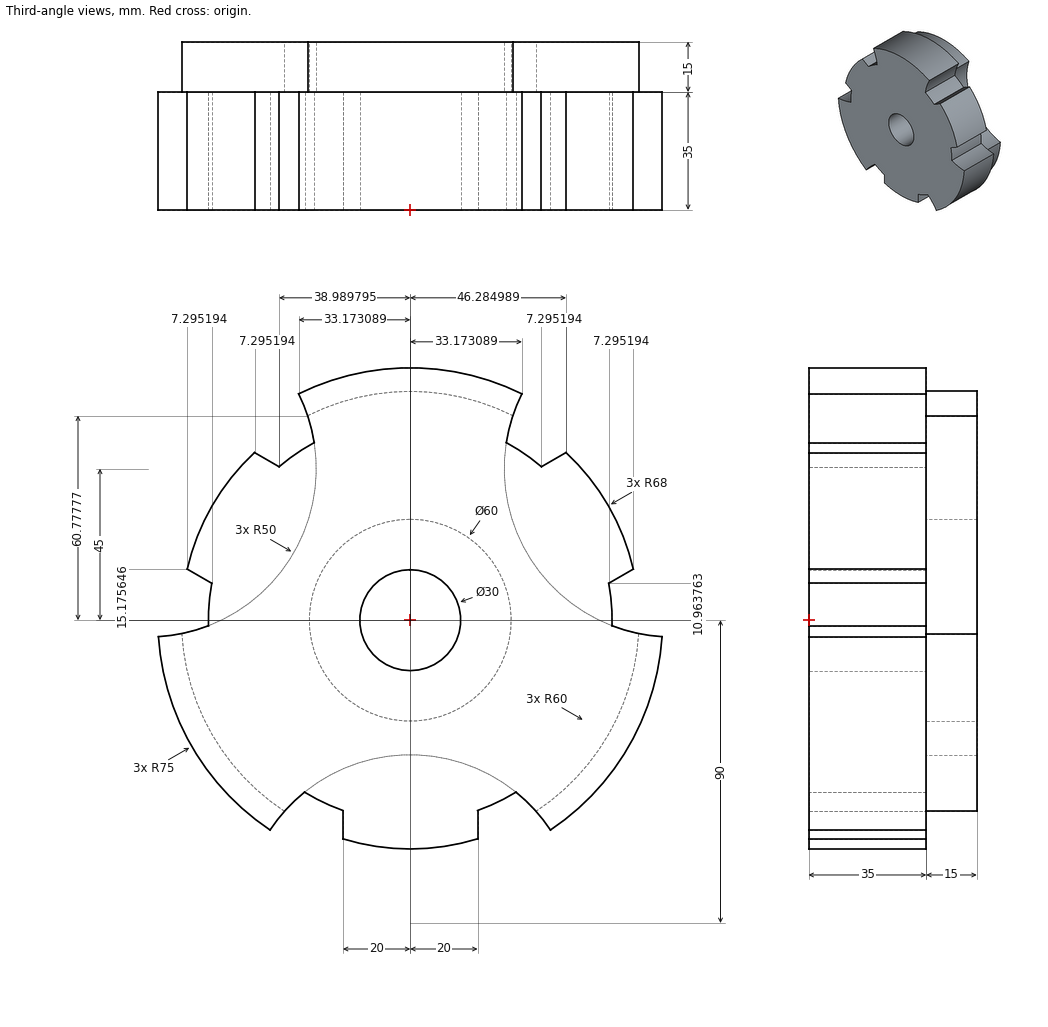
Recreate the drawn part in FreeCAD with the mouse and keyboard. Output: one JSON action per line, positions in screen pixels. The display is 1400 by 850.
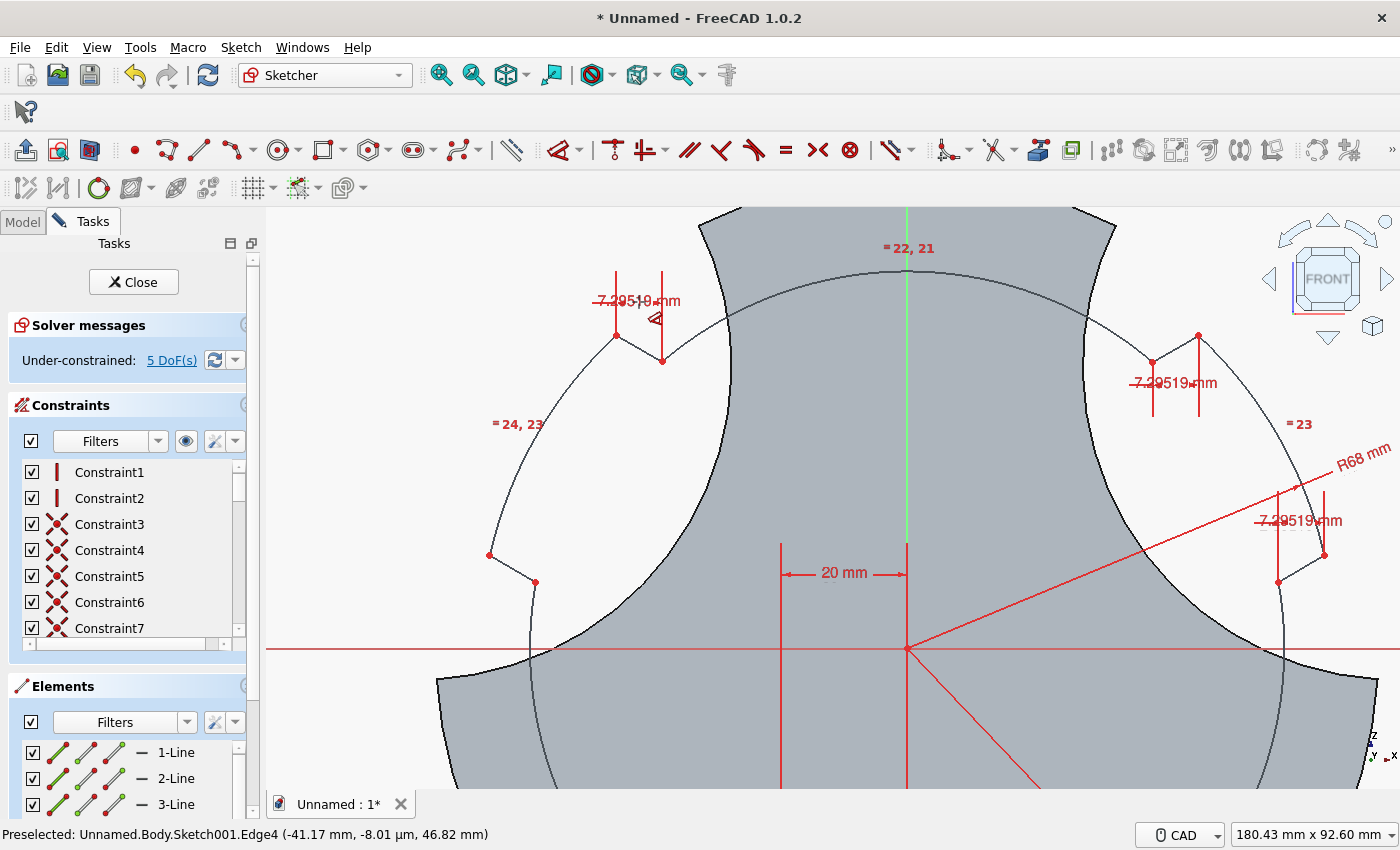
{"action": "left_click", "coordinate": [504, 564]}
{"action": "left_click", "coordinate": [513, 522]}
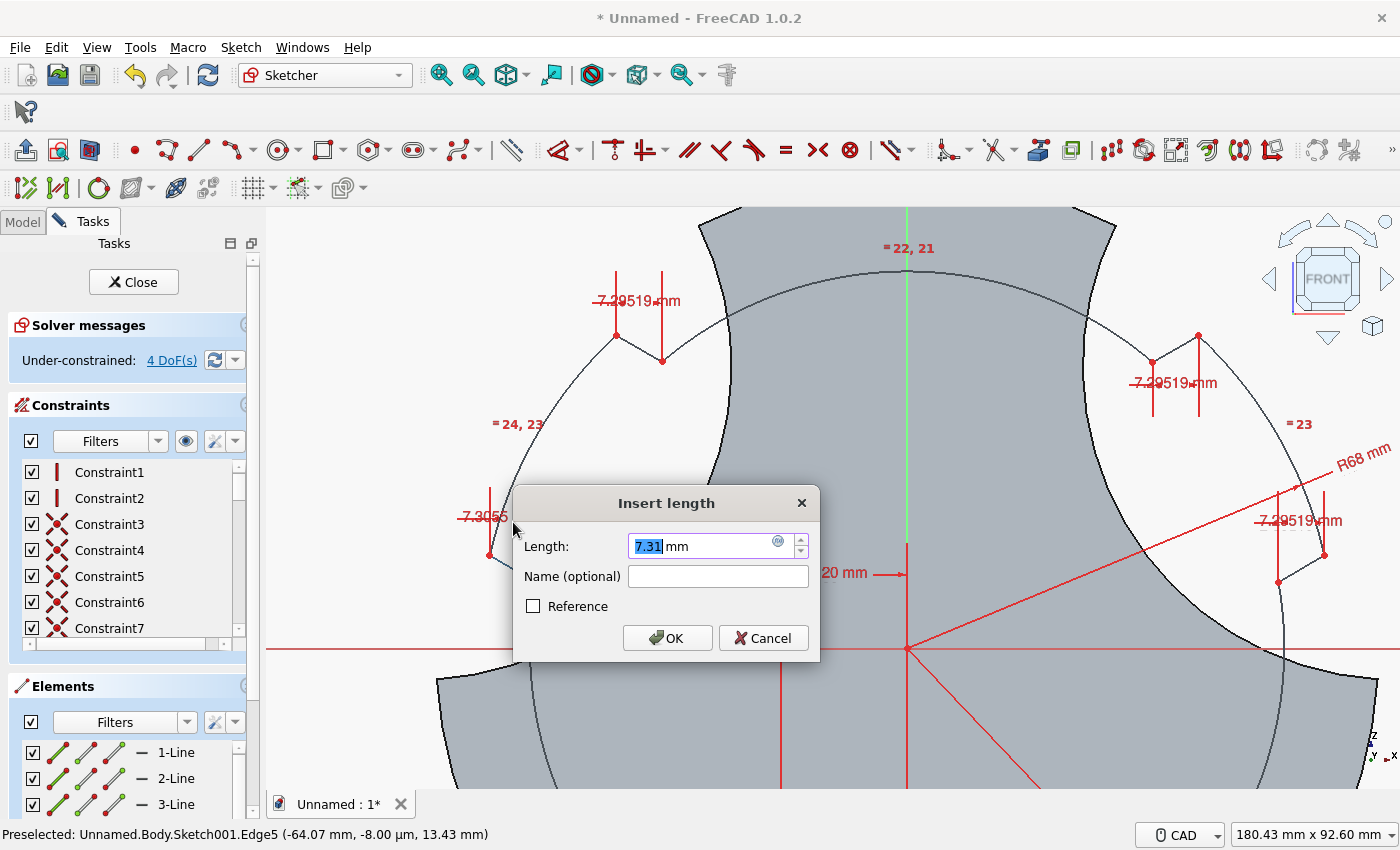
{"action": "type", "text": "7.295194"}
{"action": "key", "text": "Return"}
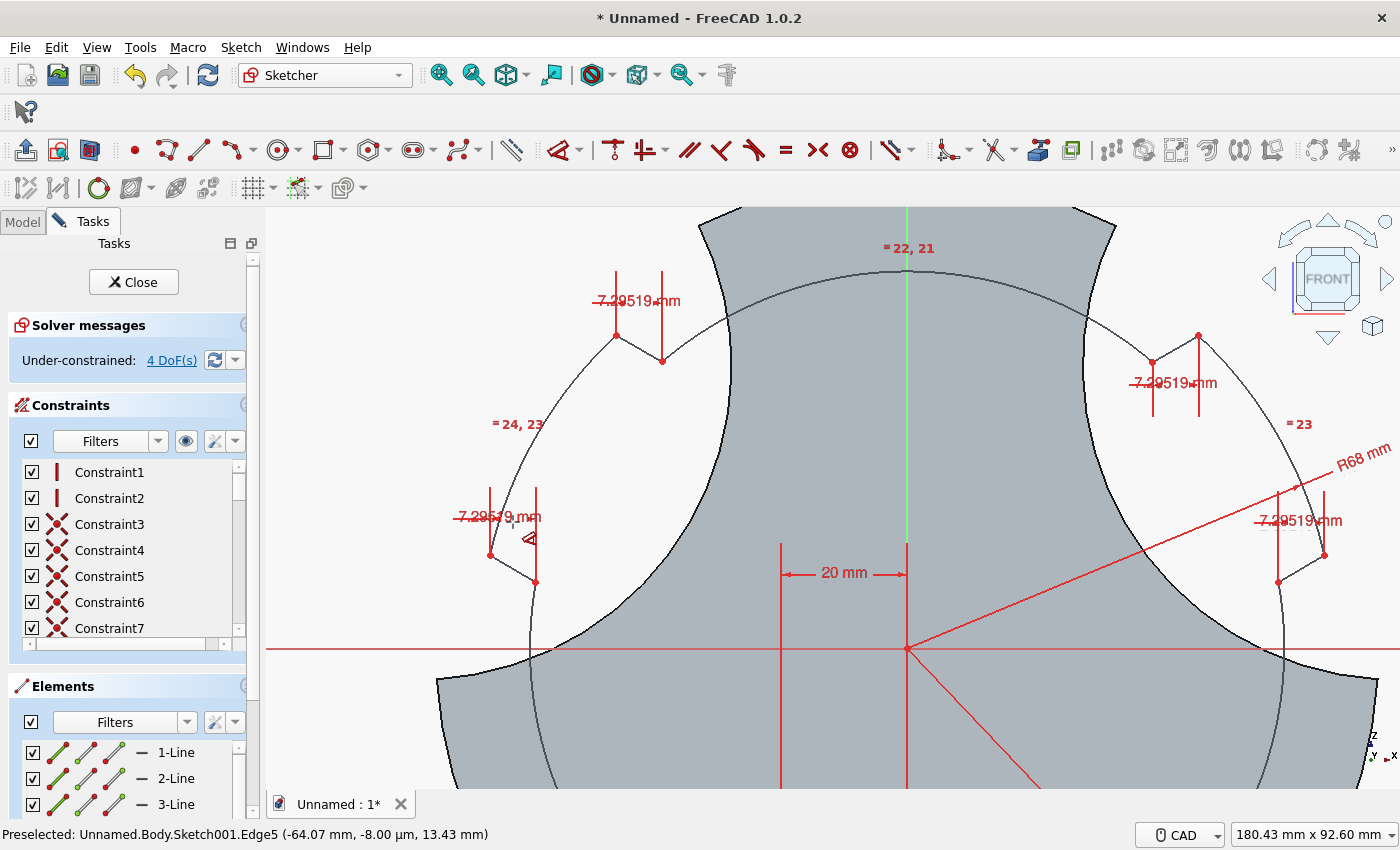
{"action": "scroll", "coordinate": [648, 355], "scroll_direction": "down", "scroll_amount": 4}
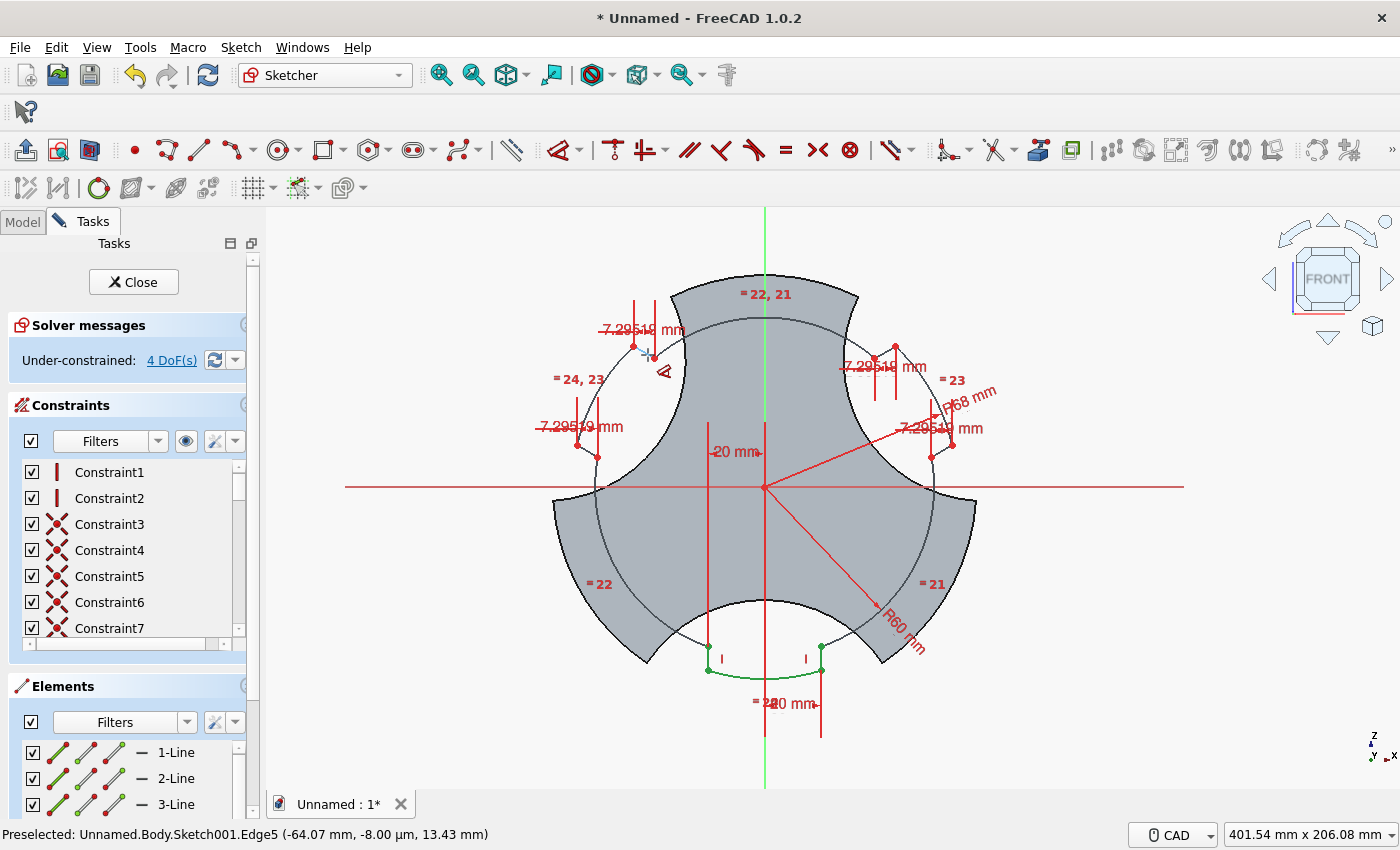
{"action": "scroll", "coordinate": [931, 457], "scroll_direction": "up", "scroll_amount": 2}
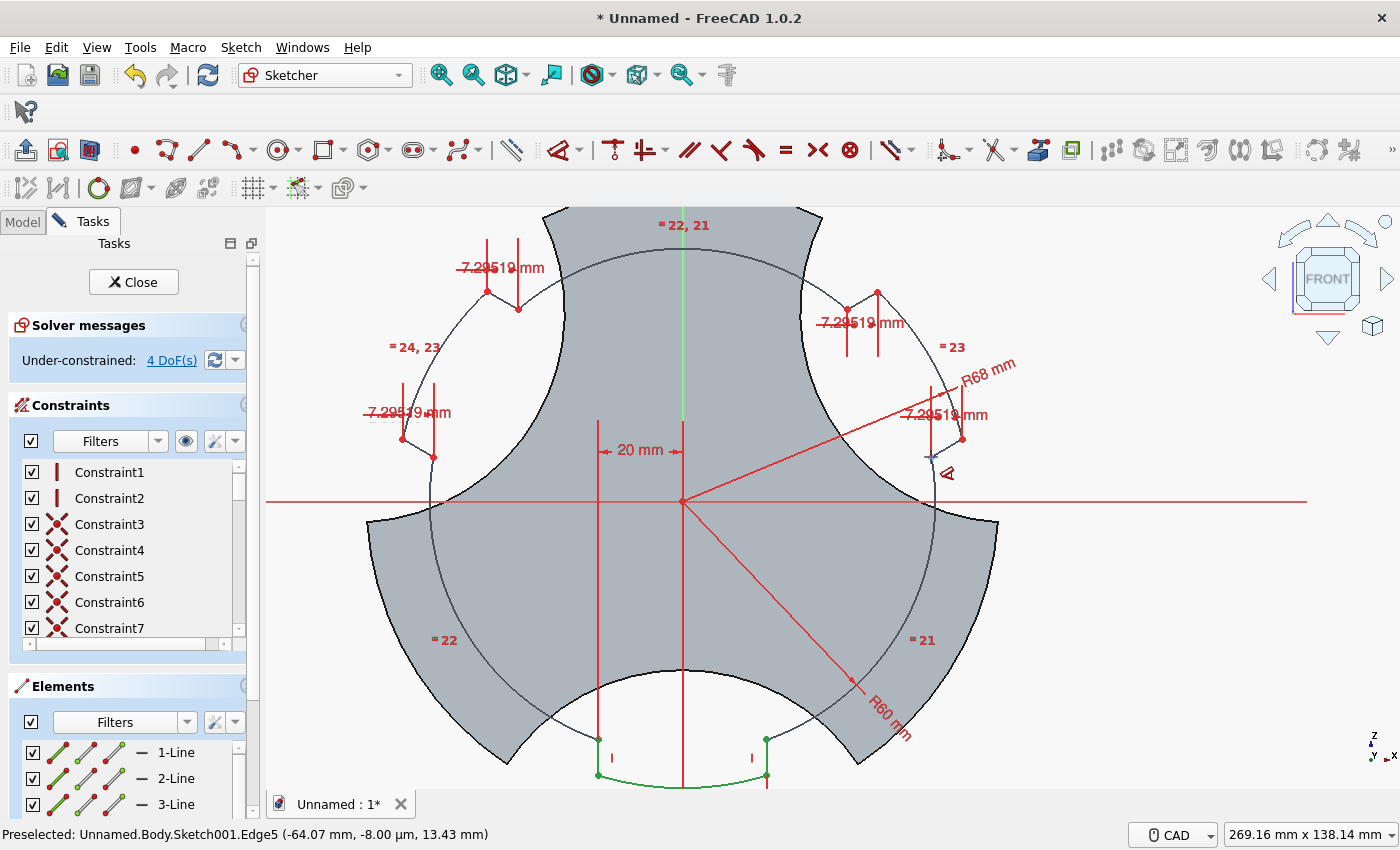
{"action": "left_click", "coordinate": [931, 457]}
{"action": "left_click", "coordinate": [965, 479]}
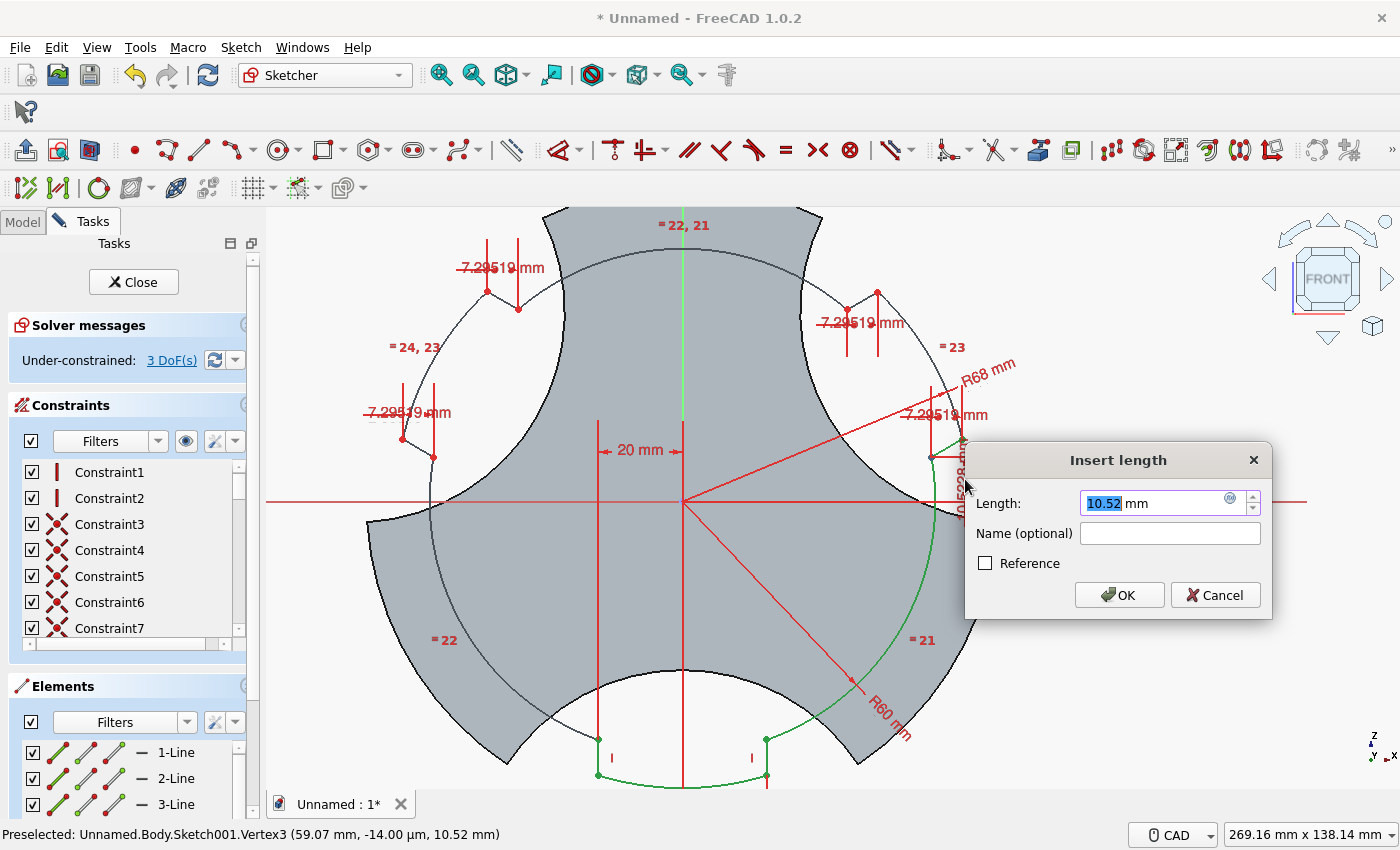
{"action": "type", "text": "10.963763"}
{"action": "key", "text": "Return"}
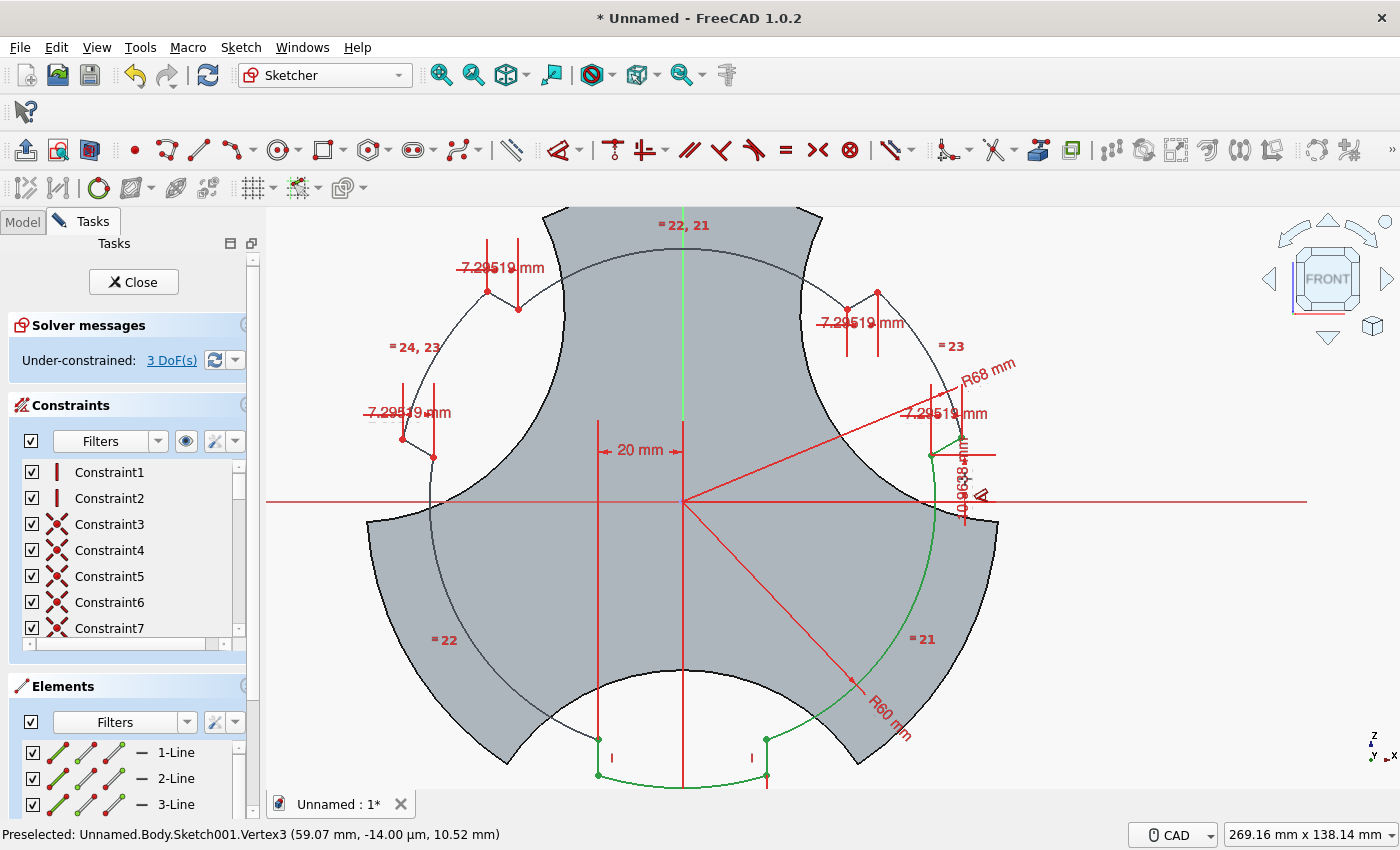
{"action": "left_click", "coordinate": [878, 292]}
{"action": "left_click", "coordinate": [825, 258]}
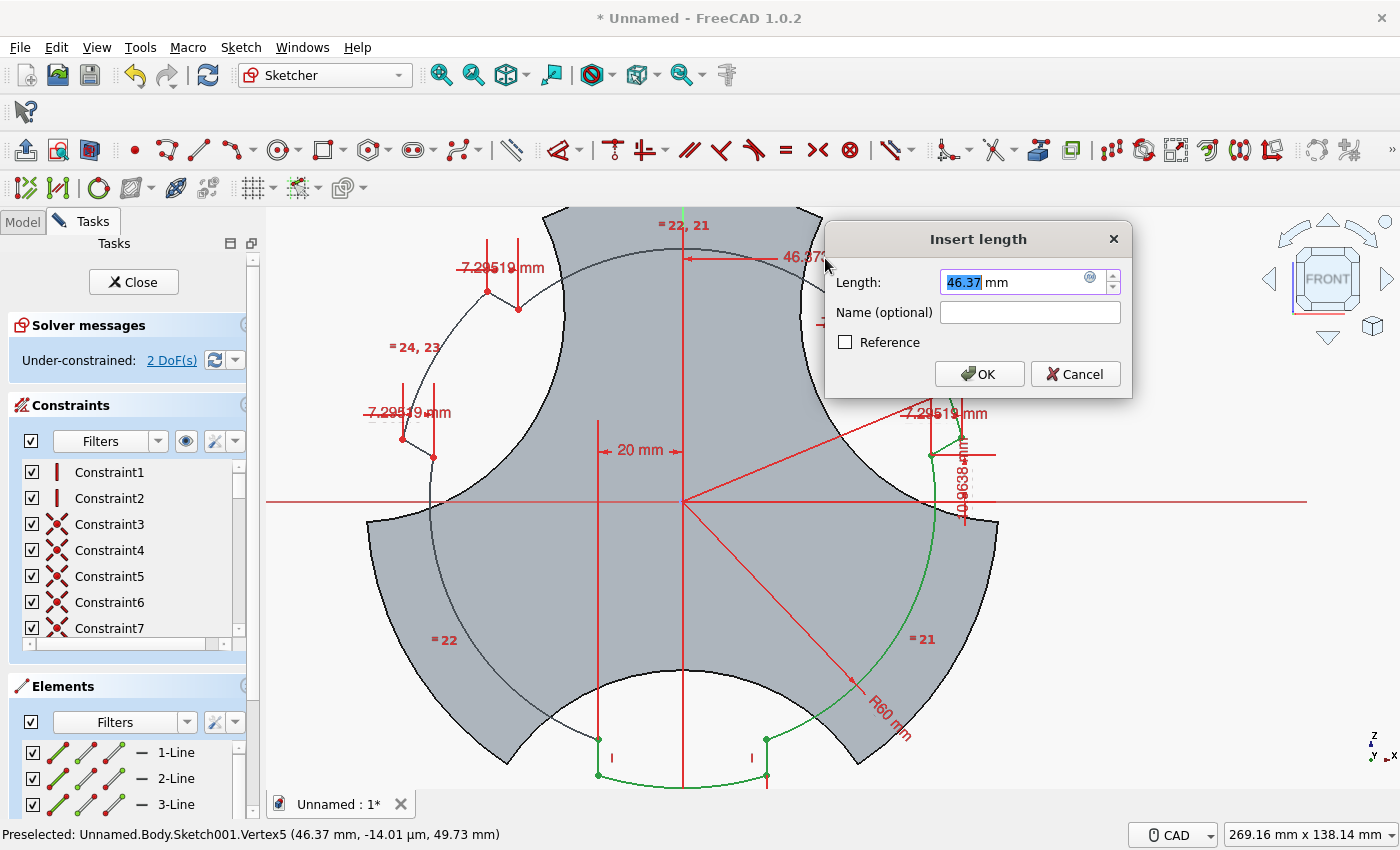
{"action": "type", "text": "46.284989"}
{"action": "key", "text": "Return"}